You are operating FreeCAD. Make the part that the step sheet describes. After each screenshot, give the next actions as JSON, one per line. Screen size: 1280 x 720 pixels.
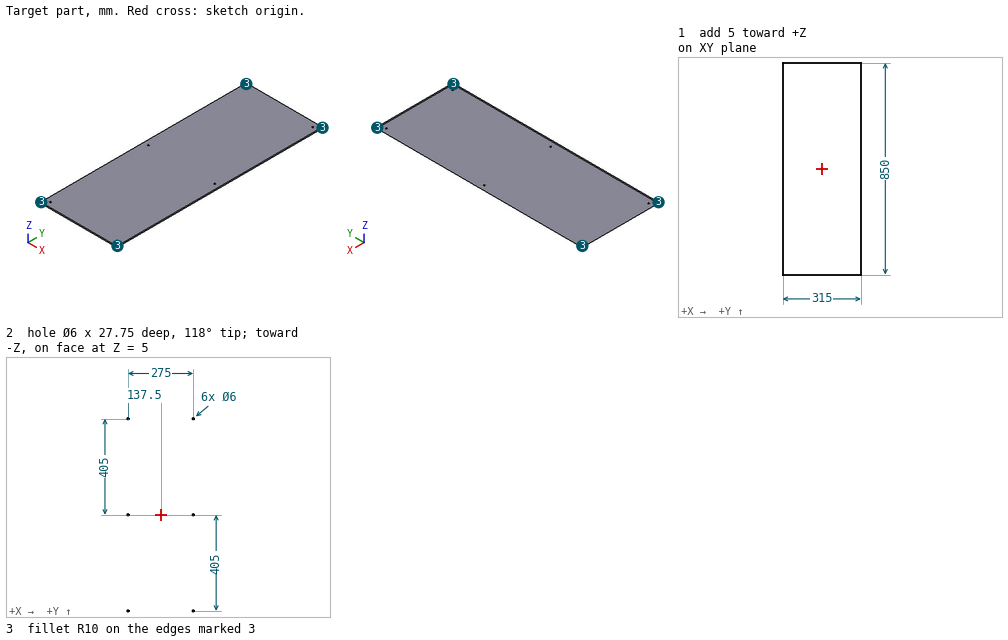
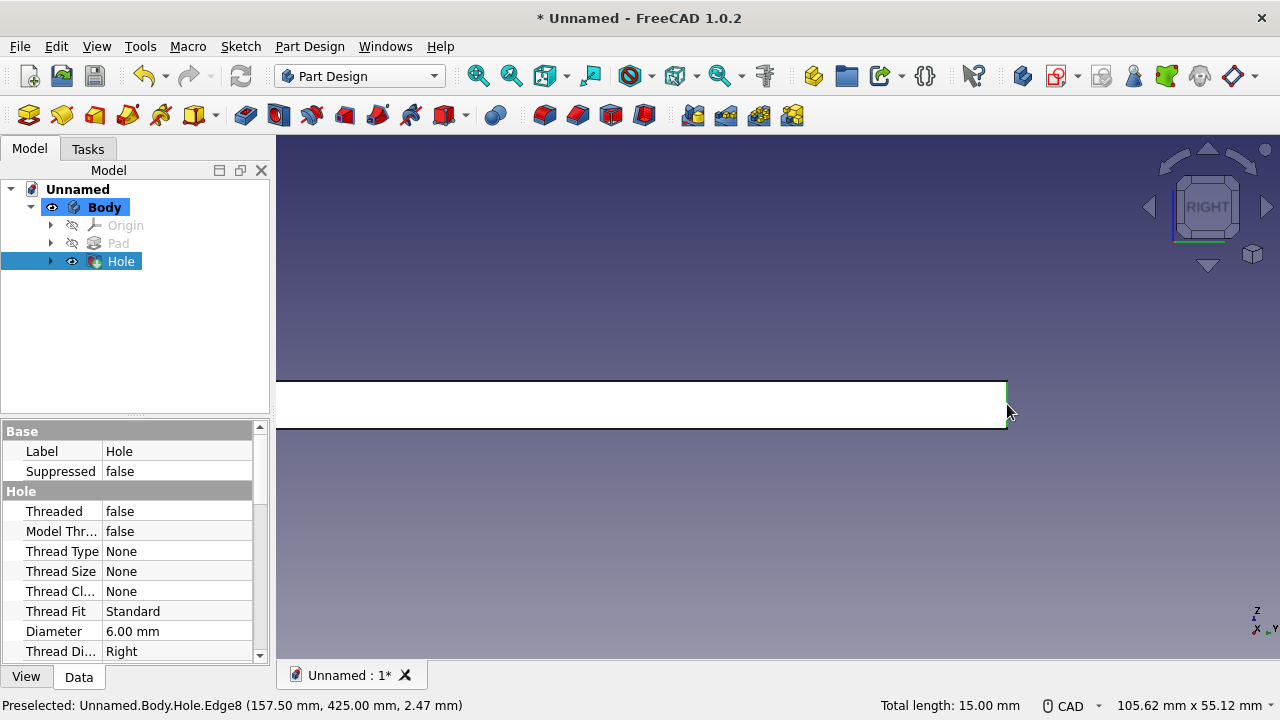
{"action": "key", "text": "v f"}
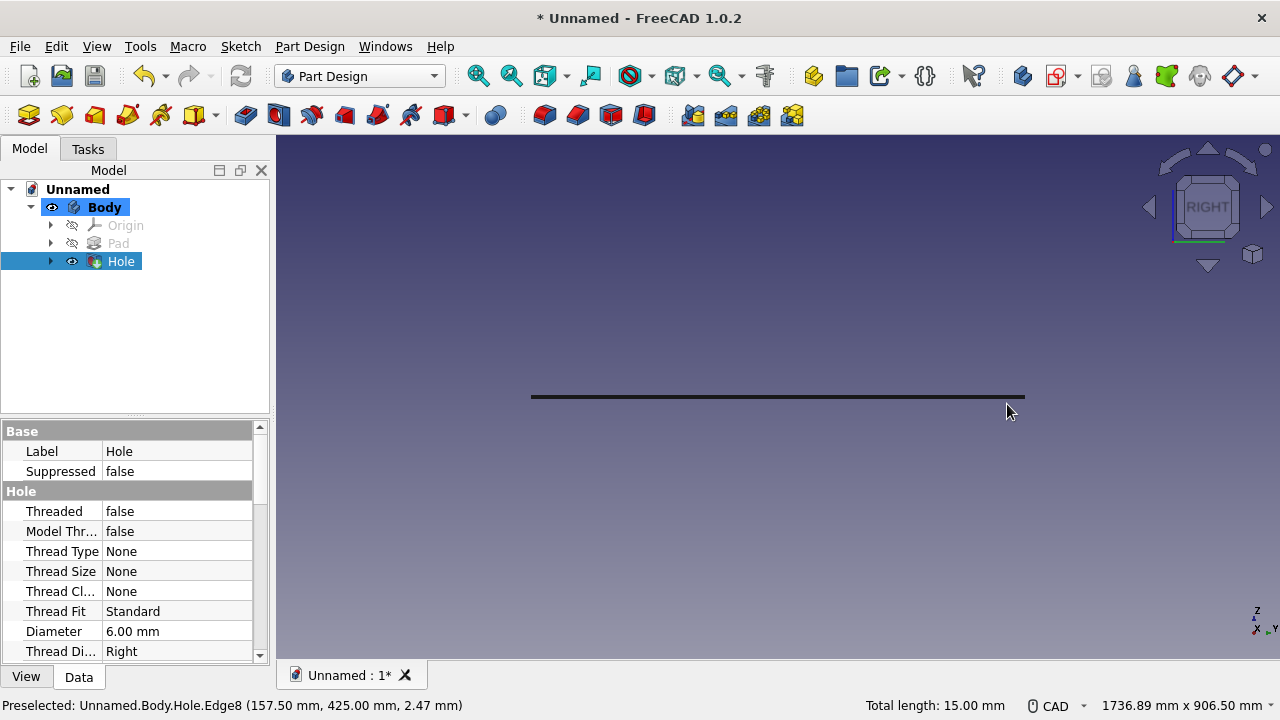
{"action": "key", "text": "5"}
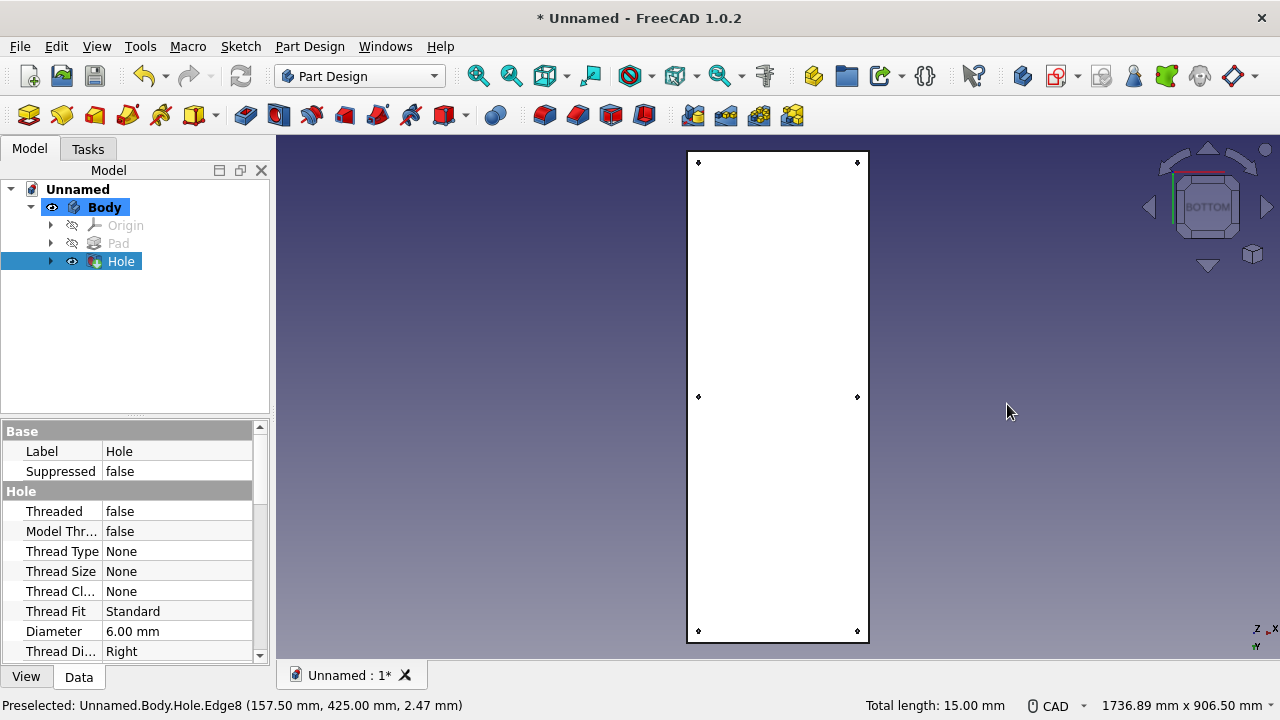
{"action": "key", "text": "4"}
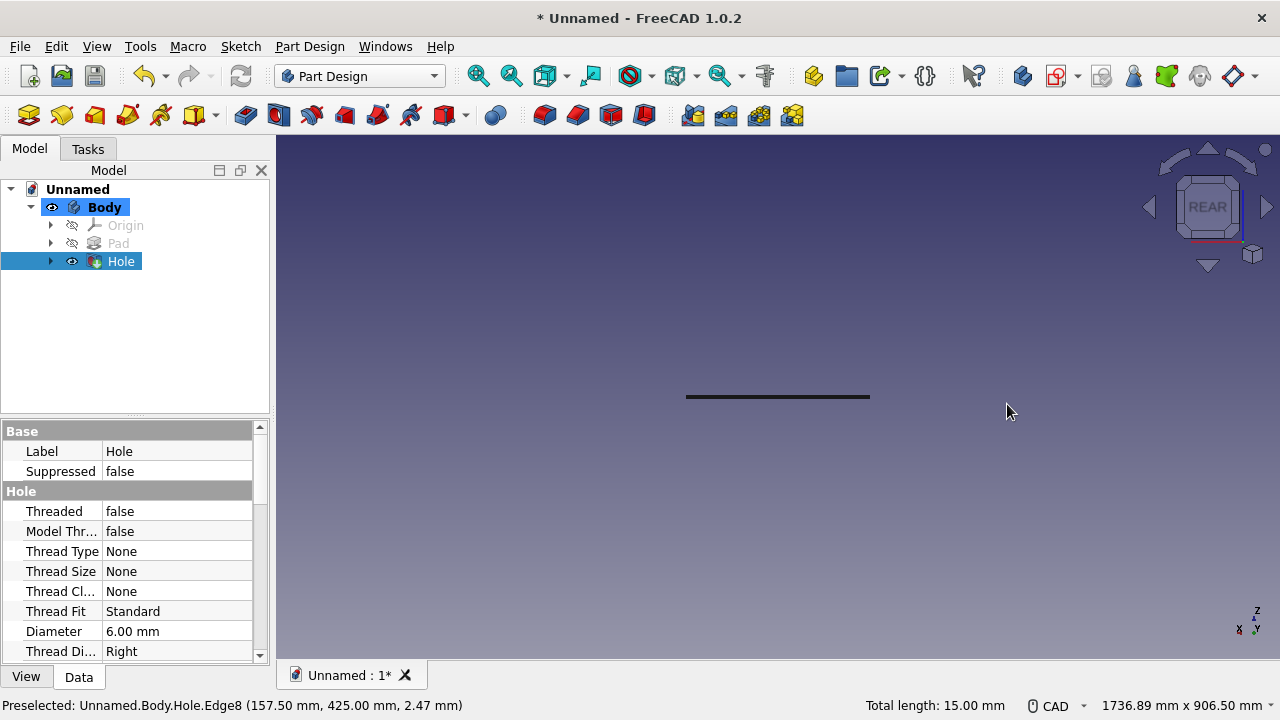
{"action": "key", "text": "v f"}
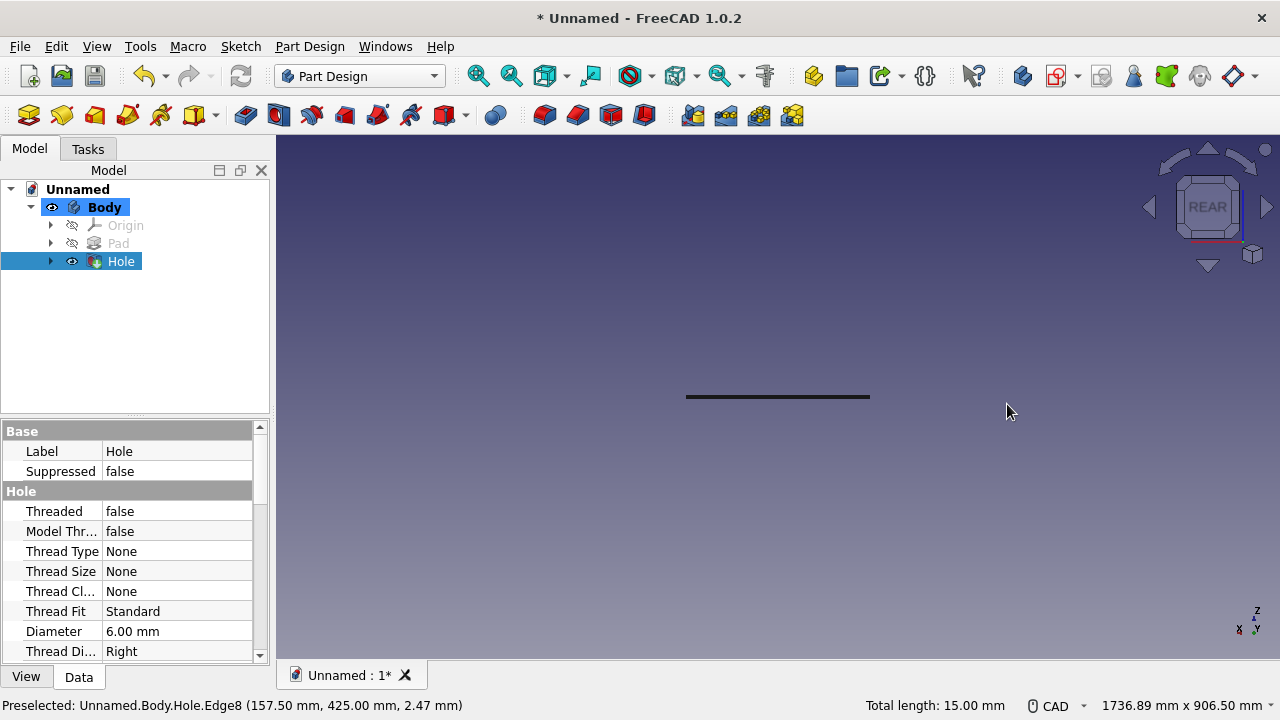
{"action": "scroll", "coordinate": [869, 396], "scroll_direction": "up", "scroll_amount": 14}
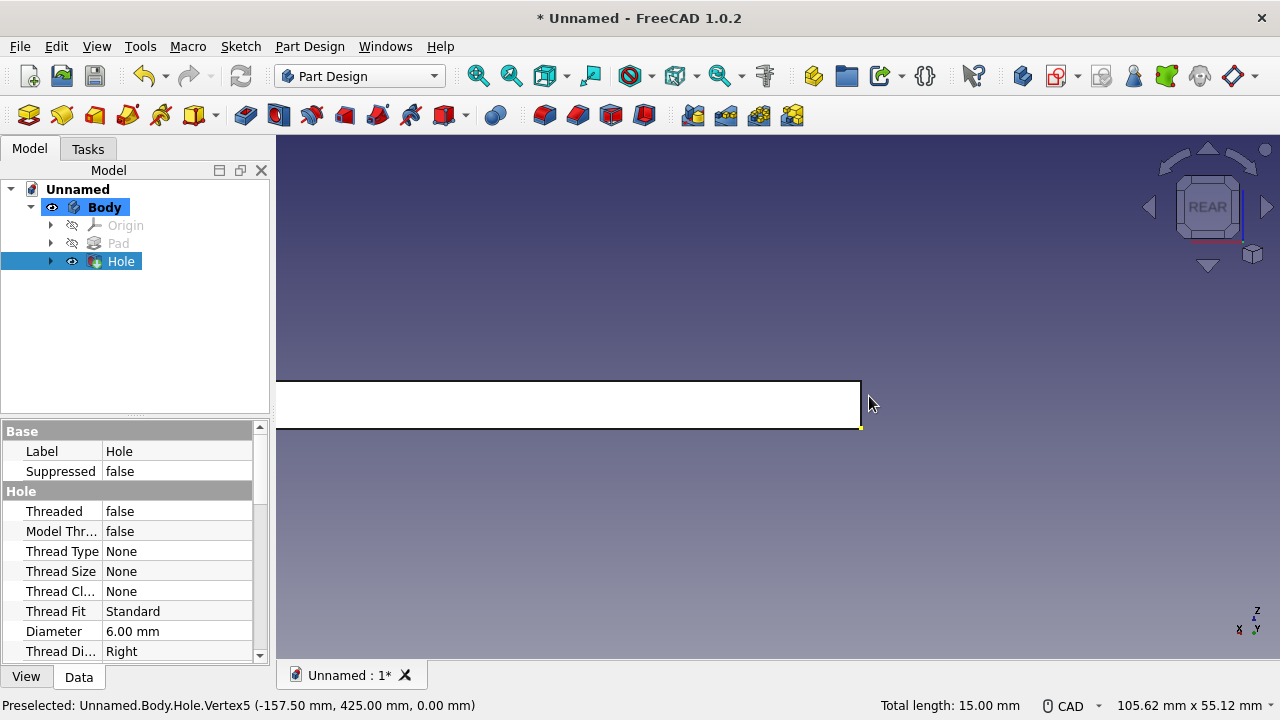
{"action": "left_click", "coordinate": [861, 404], "text": "ctrl"}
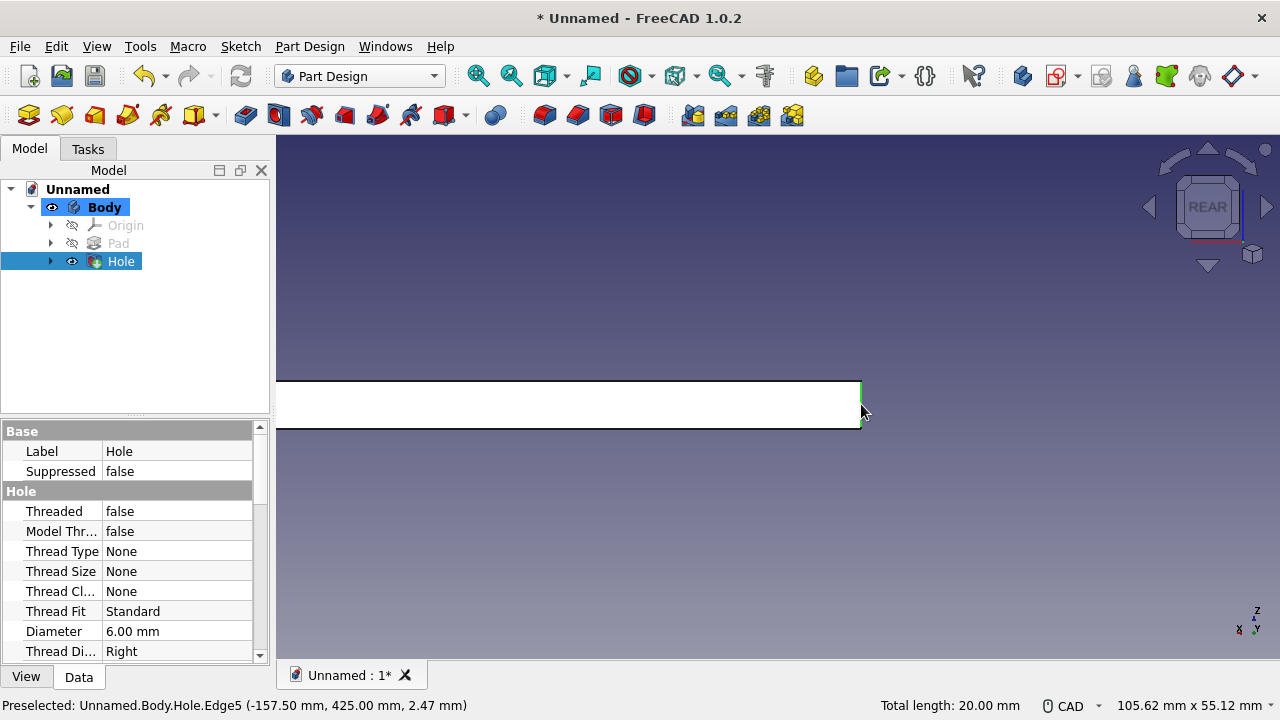
{"action": "left_click", "coordinate": [545, 116]}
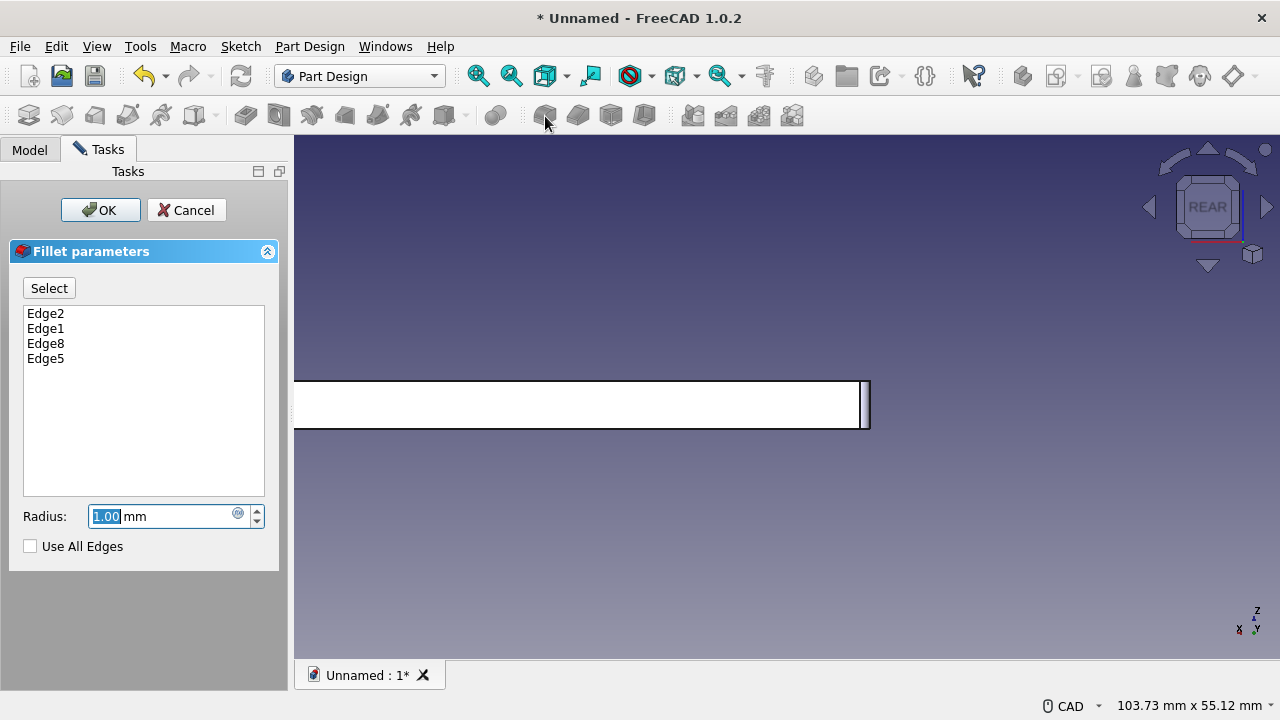
{"action": "type", "text": "10"}
{"action": "key", "text": "Tab"}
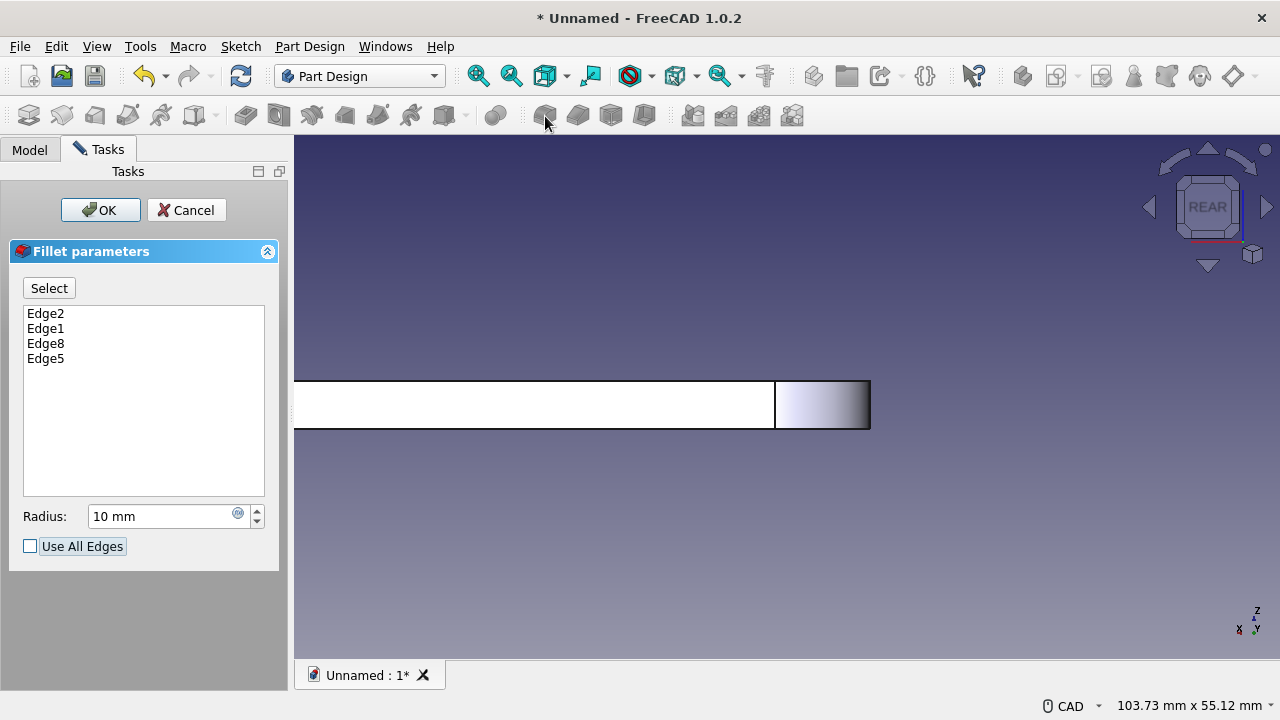
{"action": "left_click", "coordinate": [101, 210]}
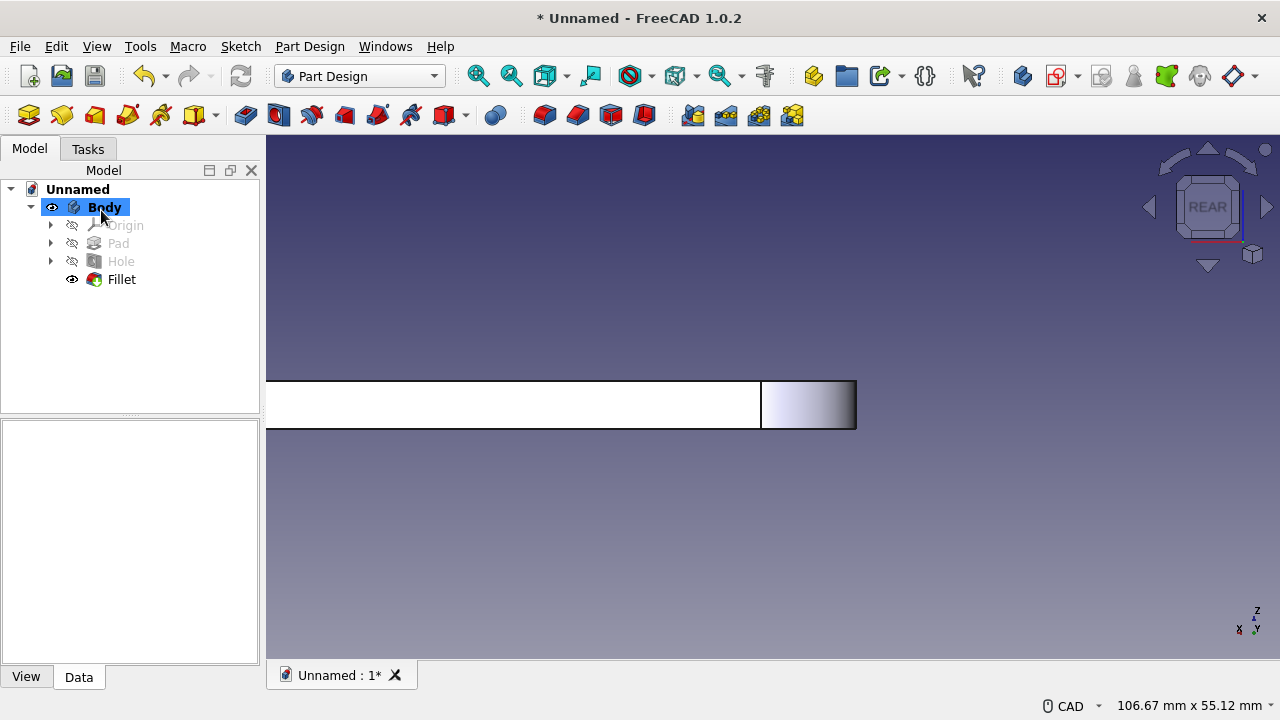
{"action": "key", "text": "0"}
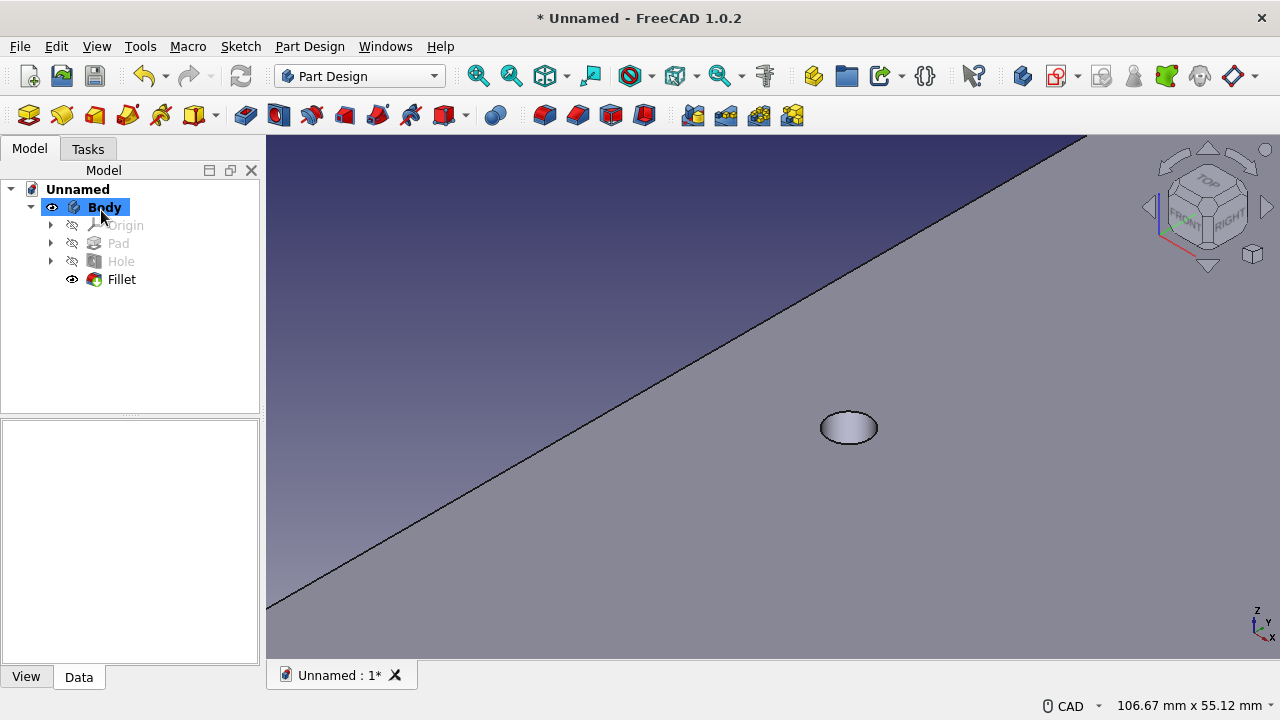
{"action": "key", "text": "v f"}